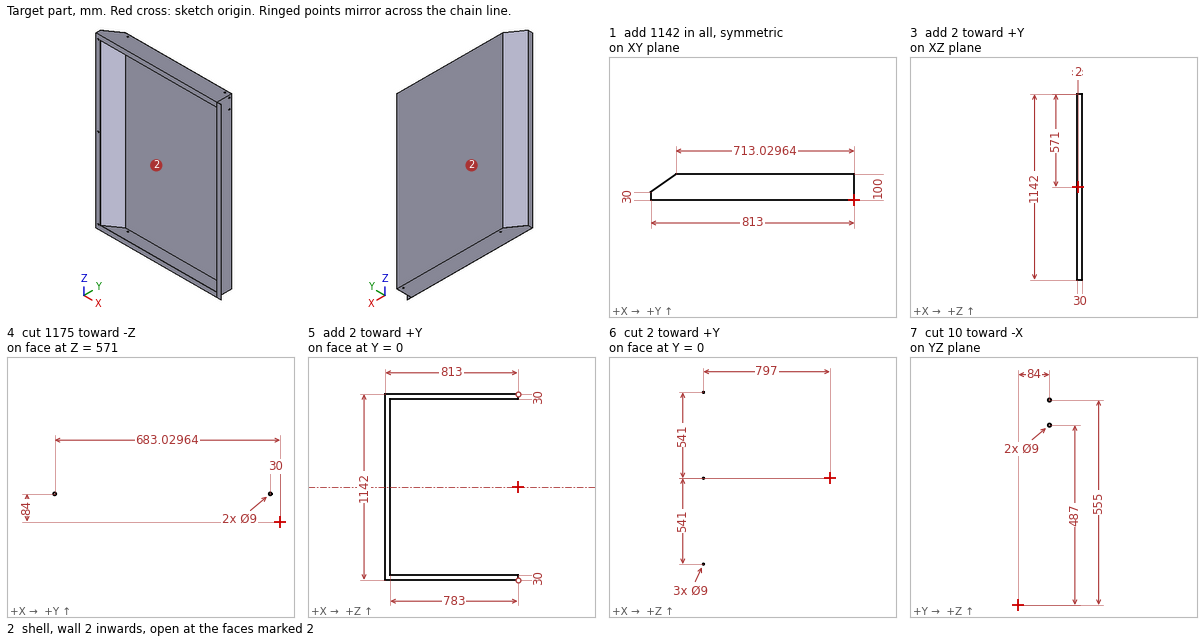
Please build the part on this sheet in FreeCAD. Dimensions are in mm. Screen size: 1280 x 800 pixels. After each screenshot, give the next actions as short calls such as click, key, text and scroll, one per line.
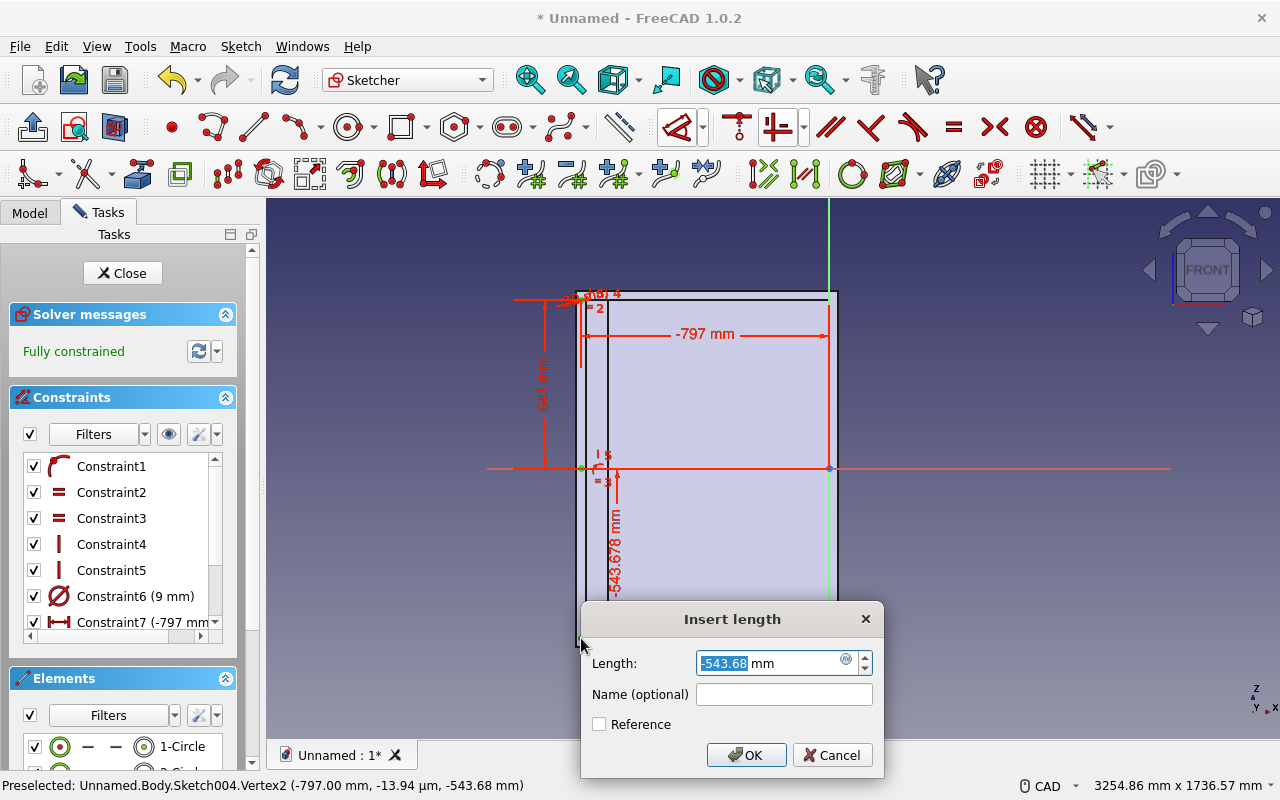
text(-541)
key(Return)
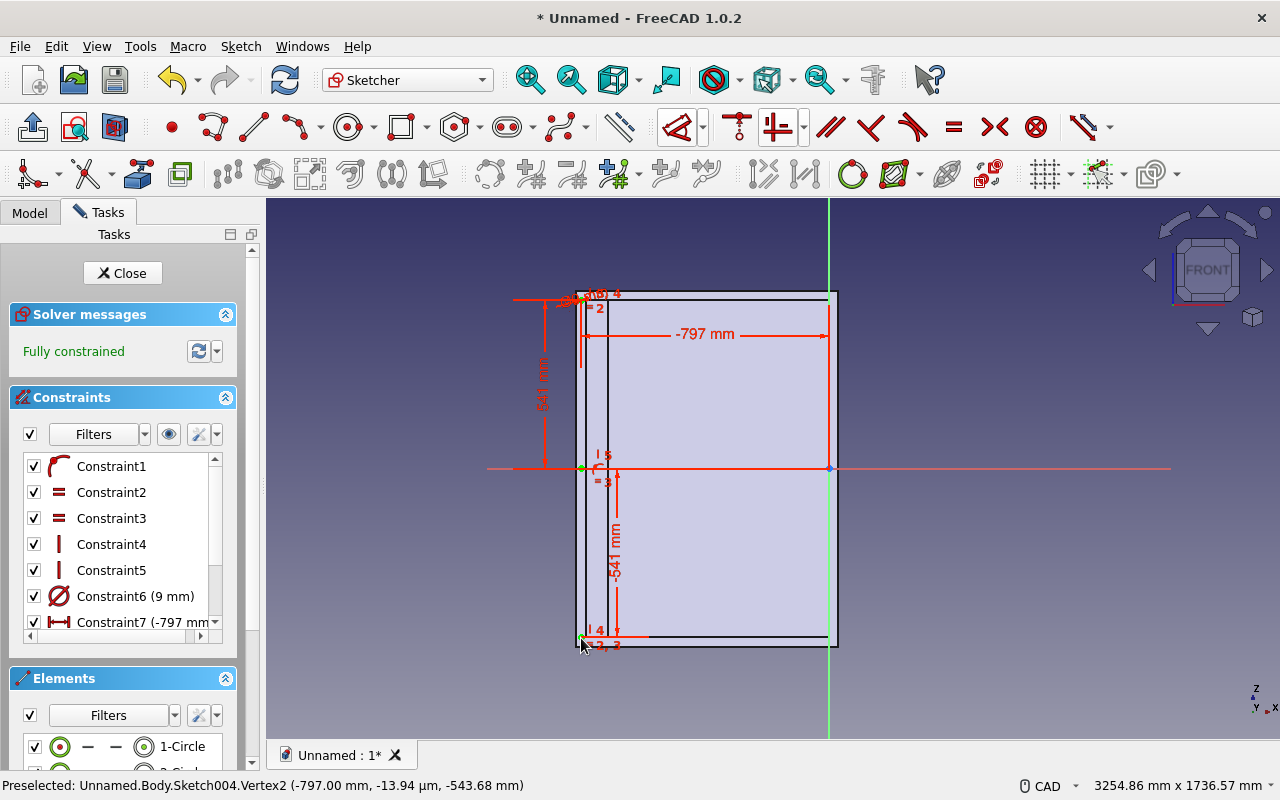
click(123, 273)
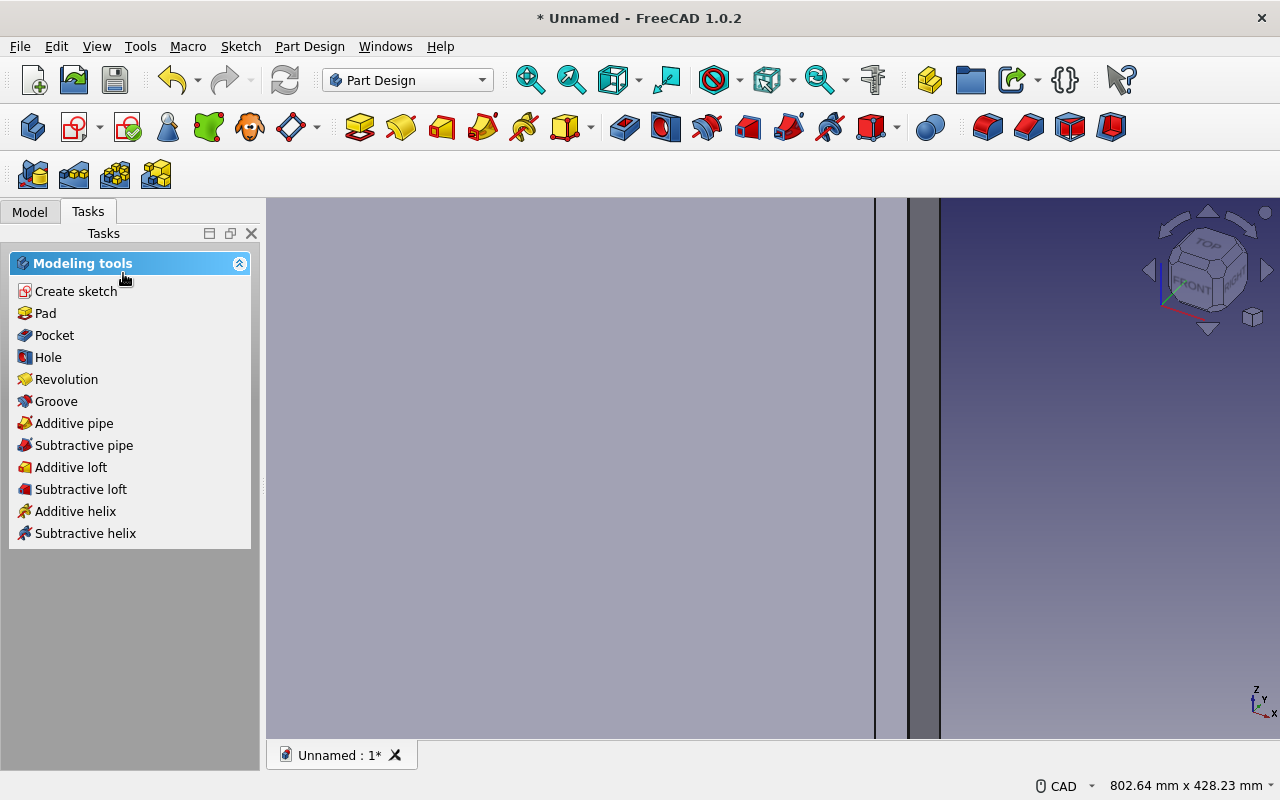
click(625, 128)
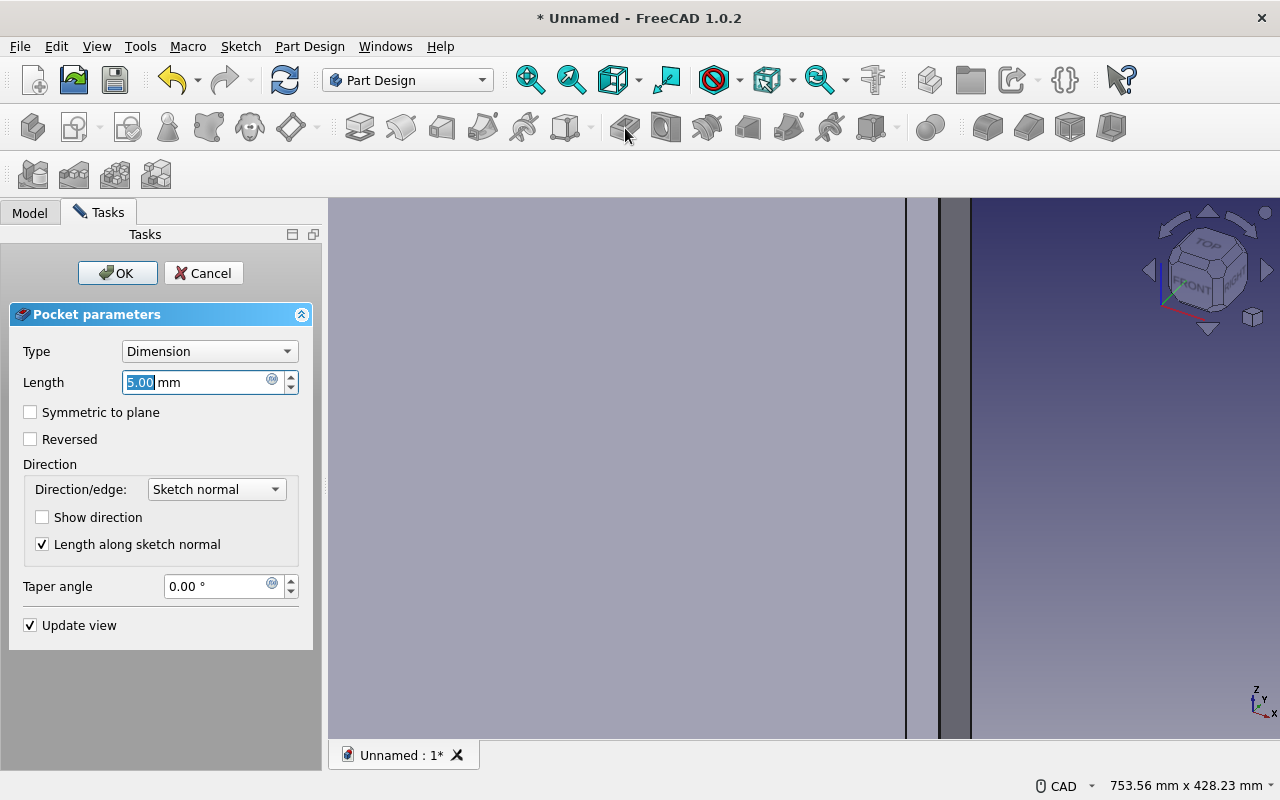
text(2)
key(Tab)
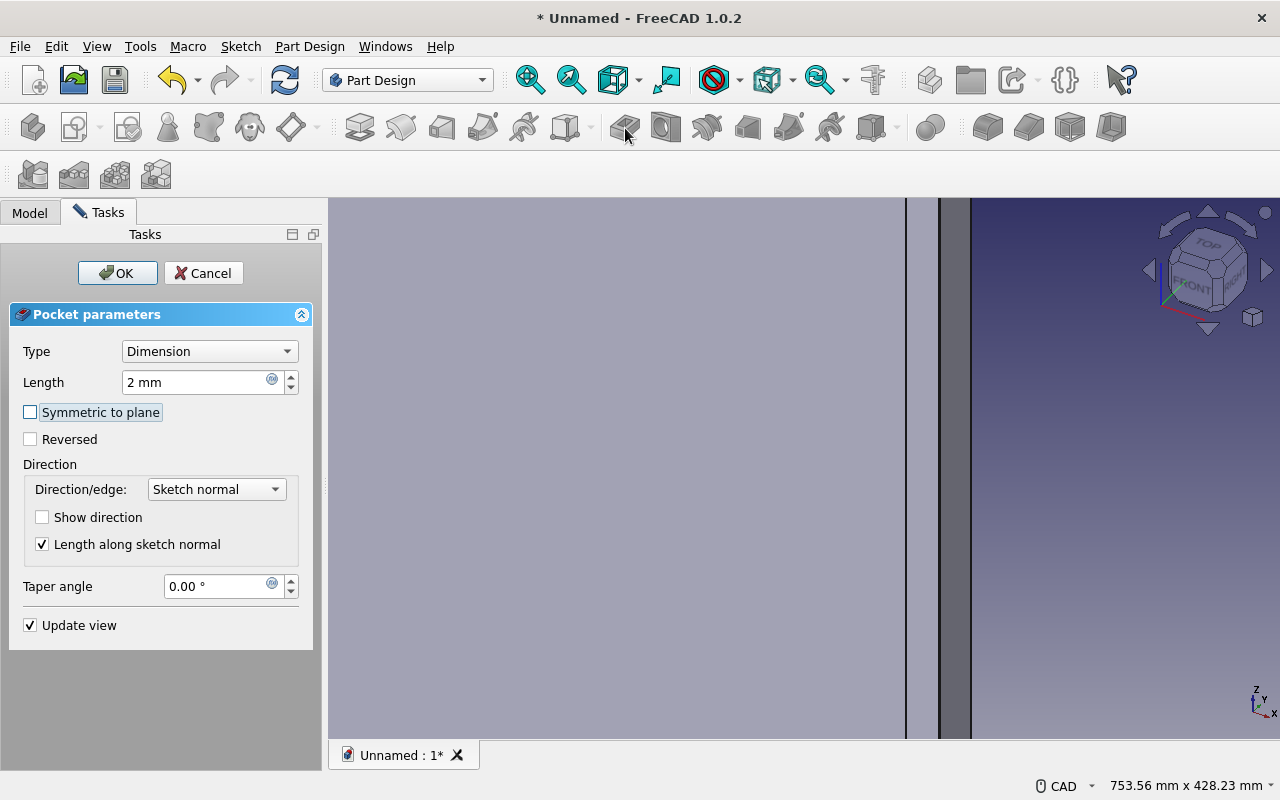
click(118, 273)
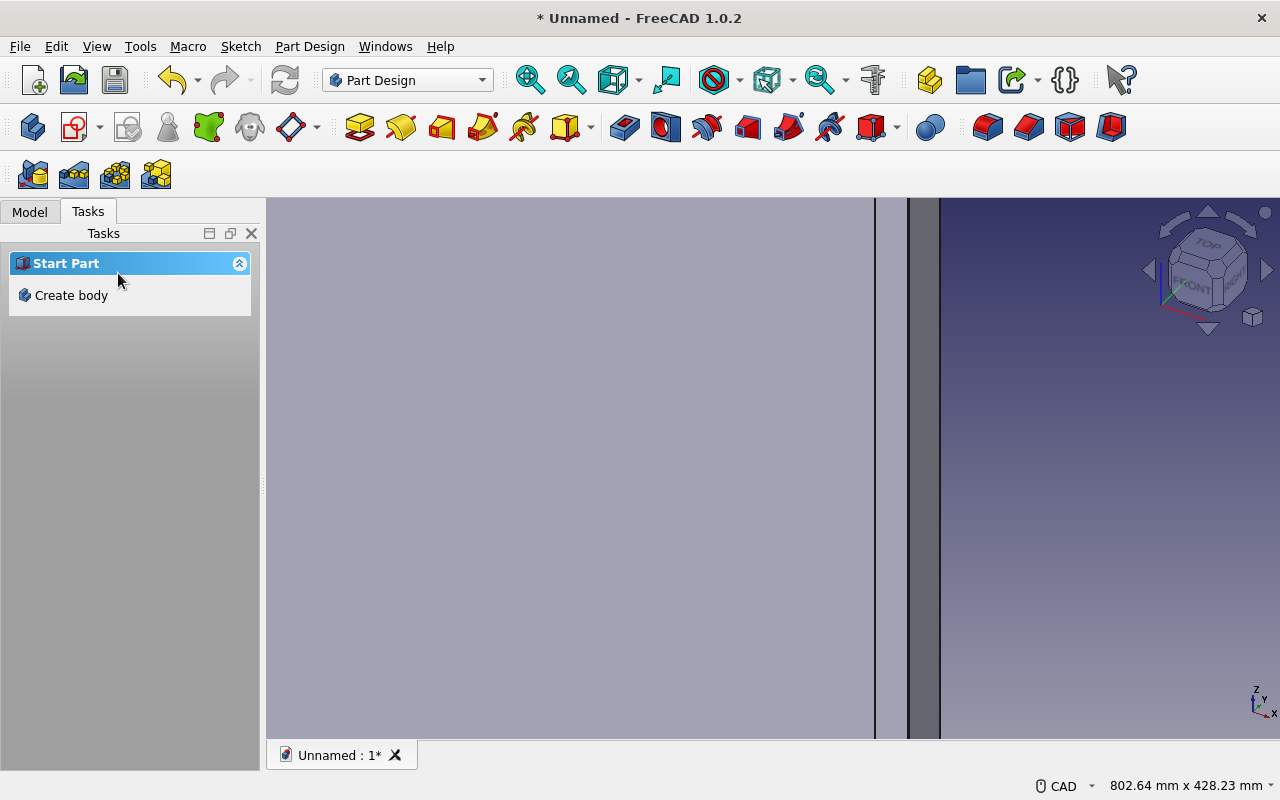
click(531, 80)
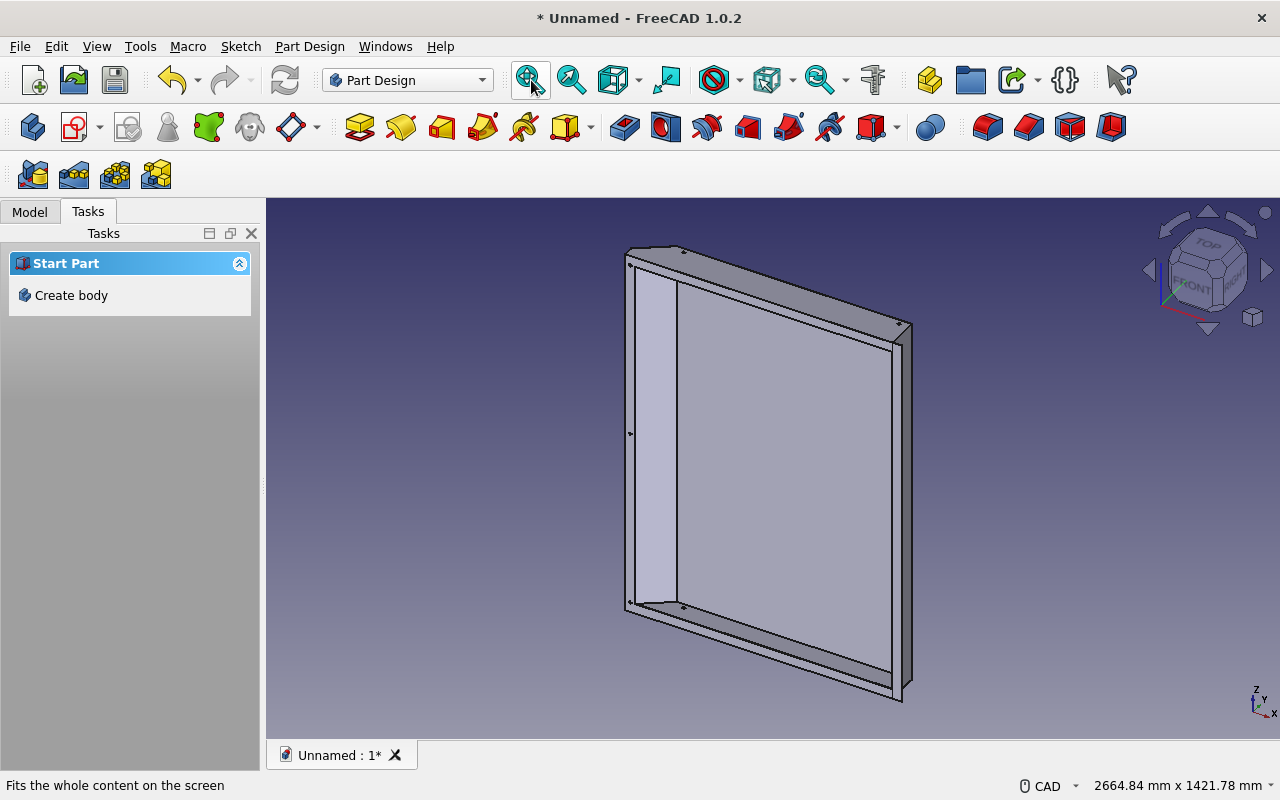
click(74, 128)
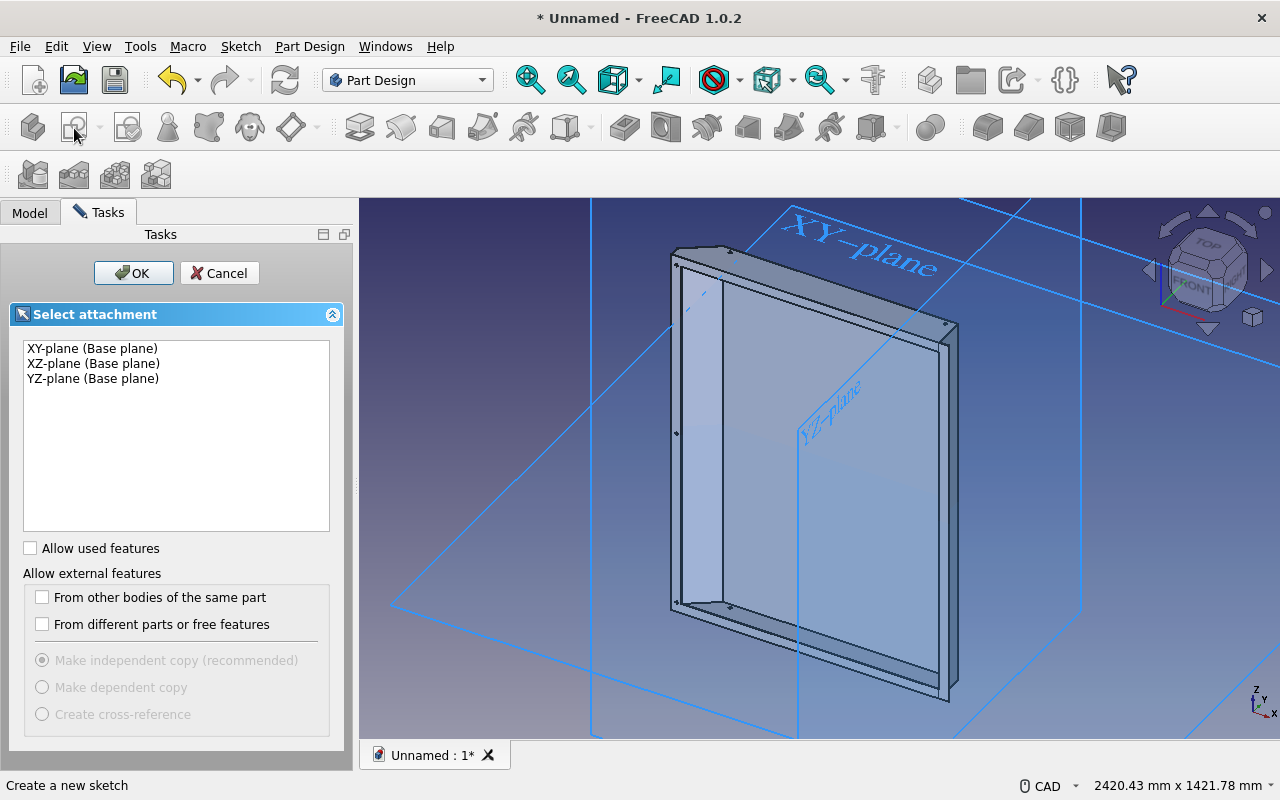
click(84, 378)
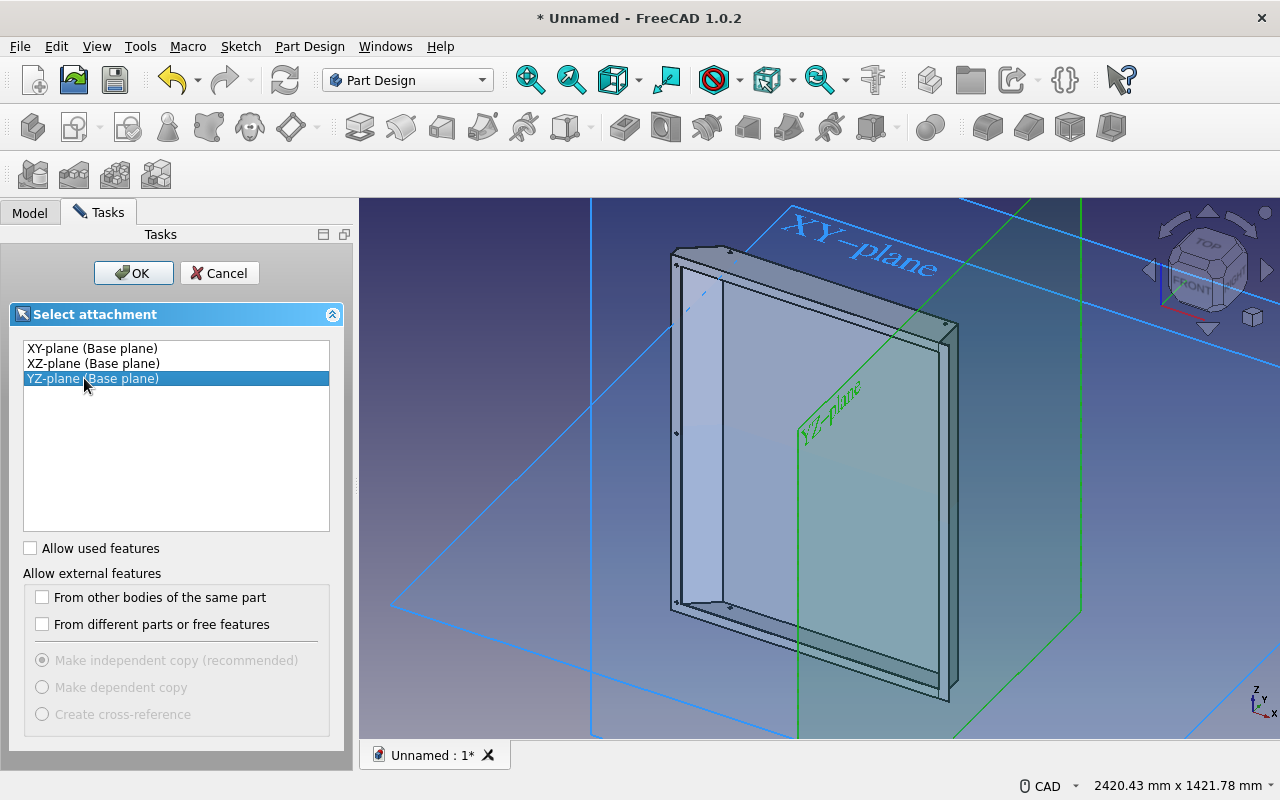
click(134, 273)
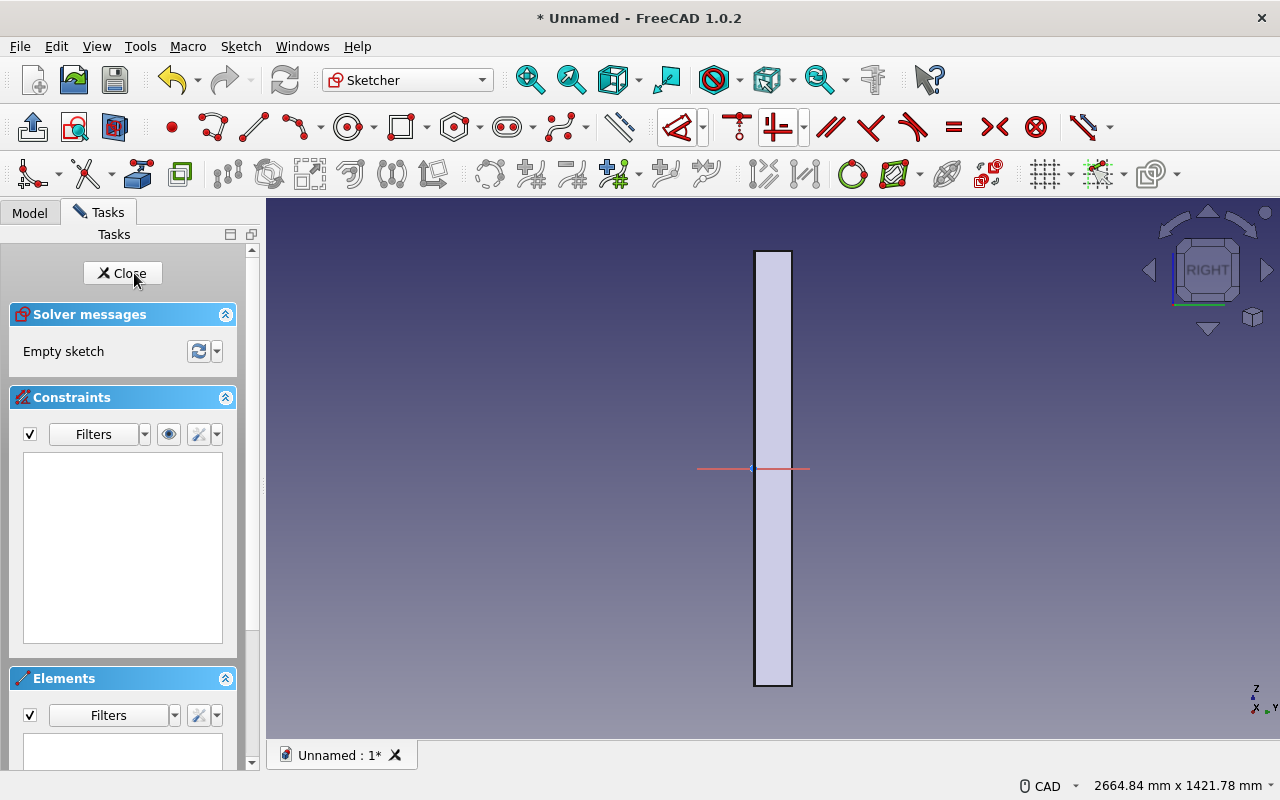
key(q)
key(s)